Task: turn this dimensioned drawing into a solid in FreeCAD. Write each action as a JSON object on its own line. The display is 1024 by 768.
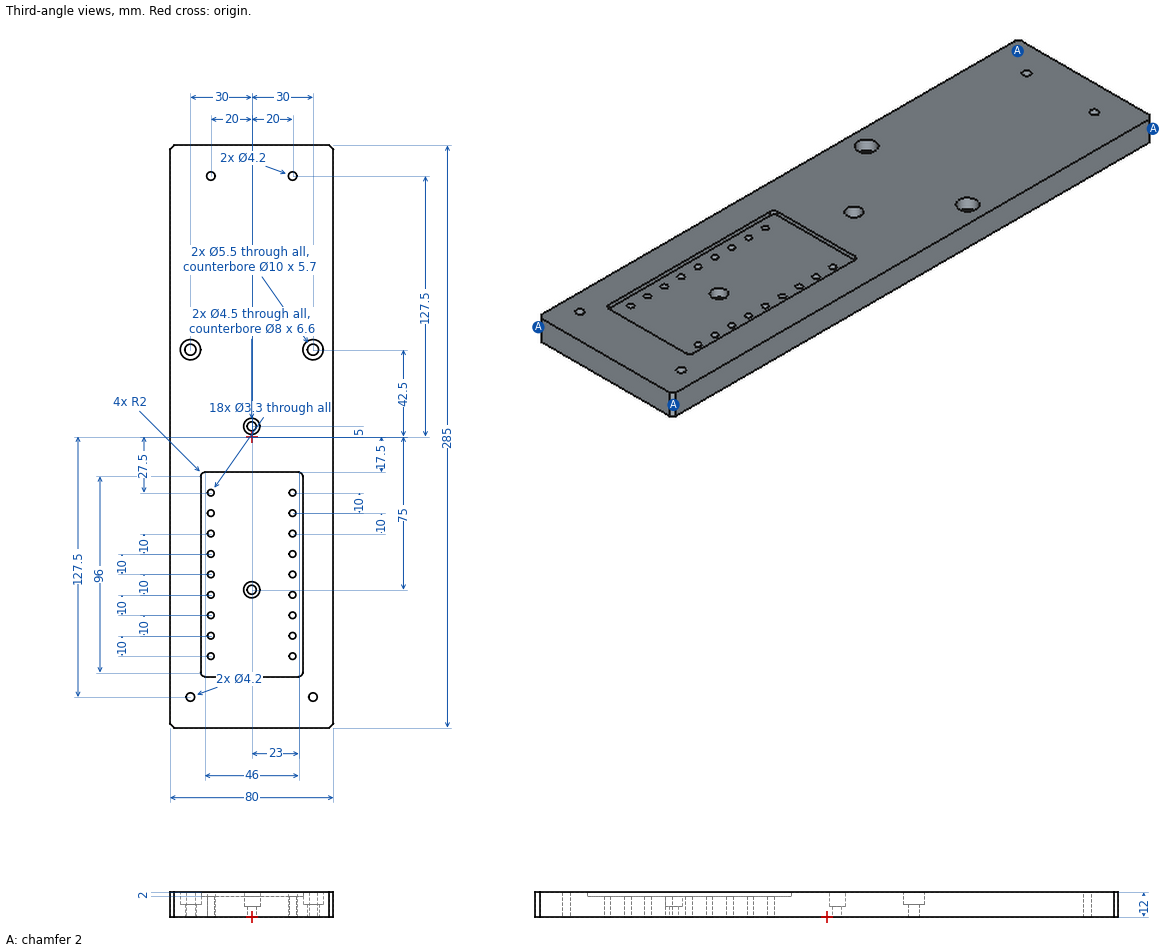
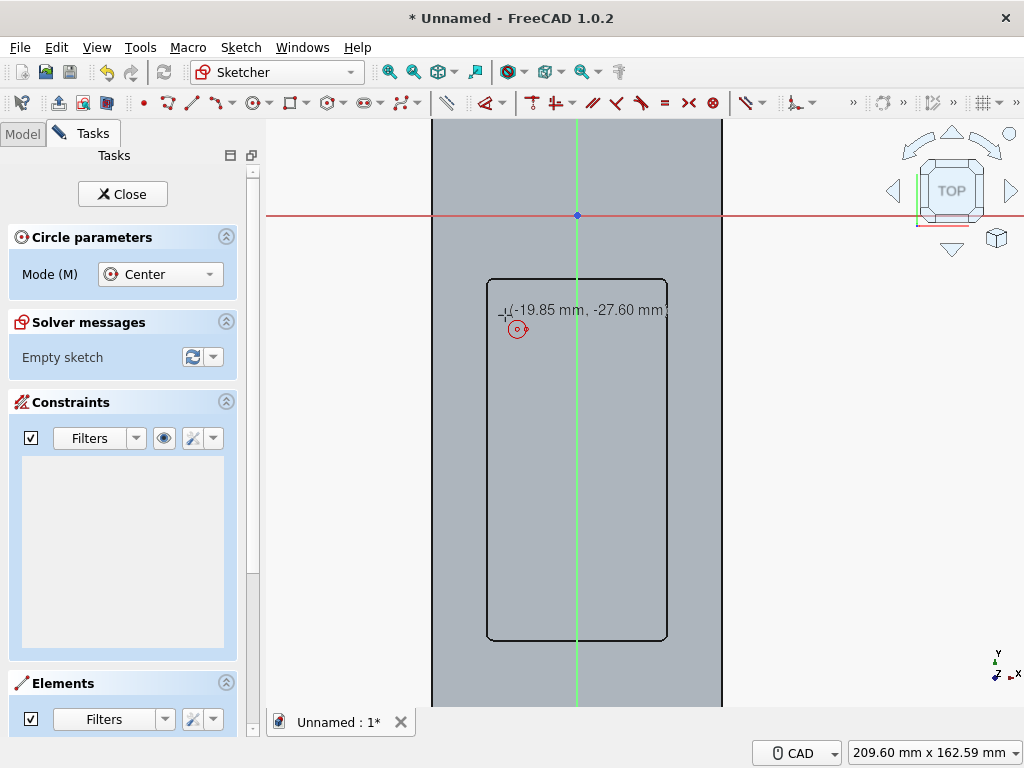
{"action": "left_click", "coordinate": [505, 315]}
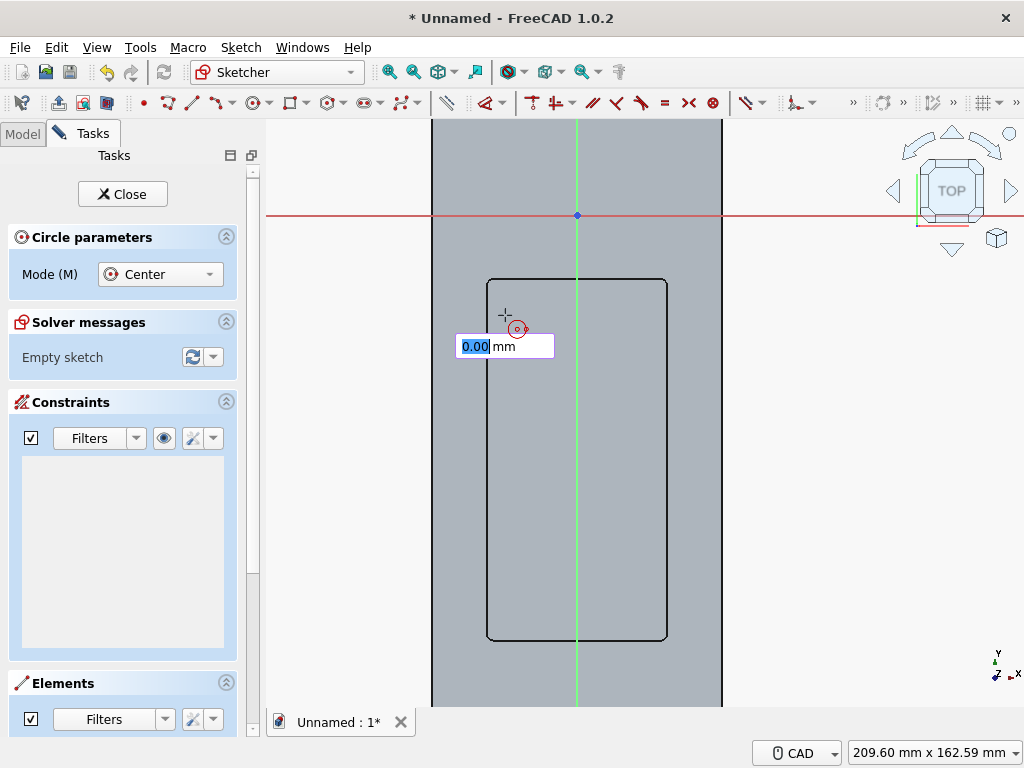
{"action": "scroll", "coordinate": [509, 311], "scroll_direction": "up", "scroll_amount": 5}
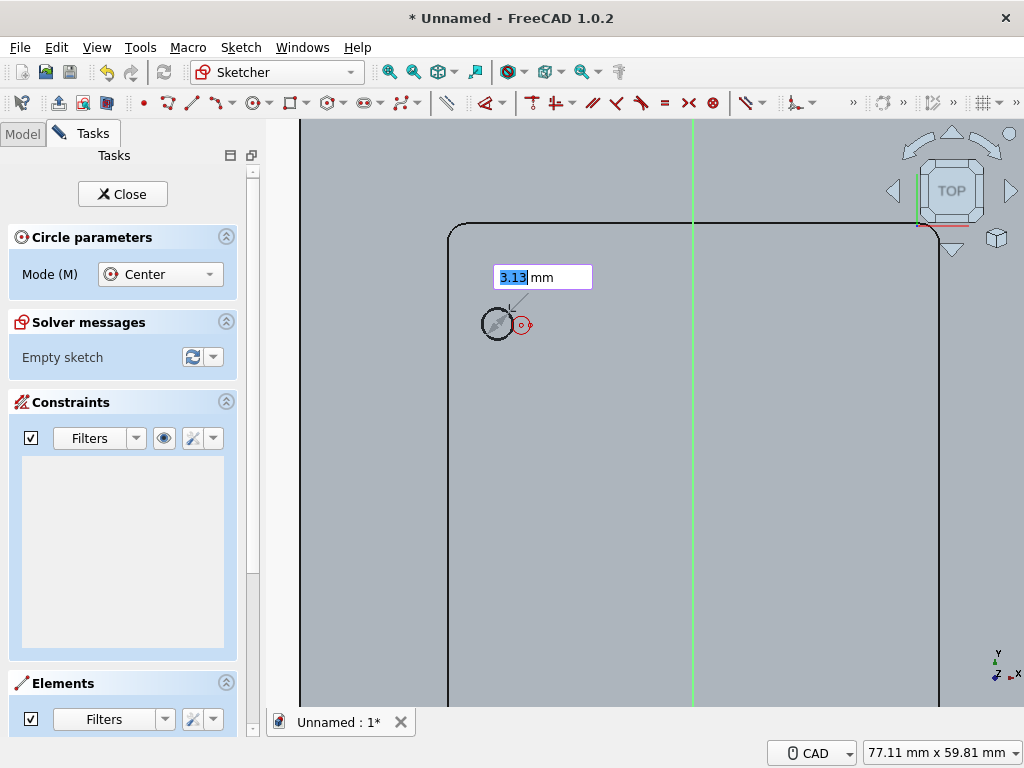
{"action": "left_click", "coordinate": [508, 310]}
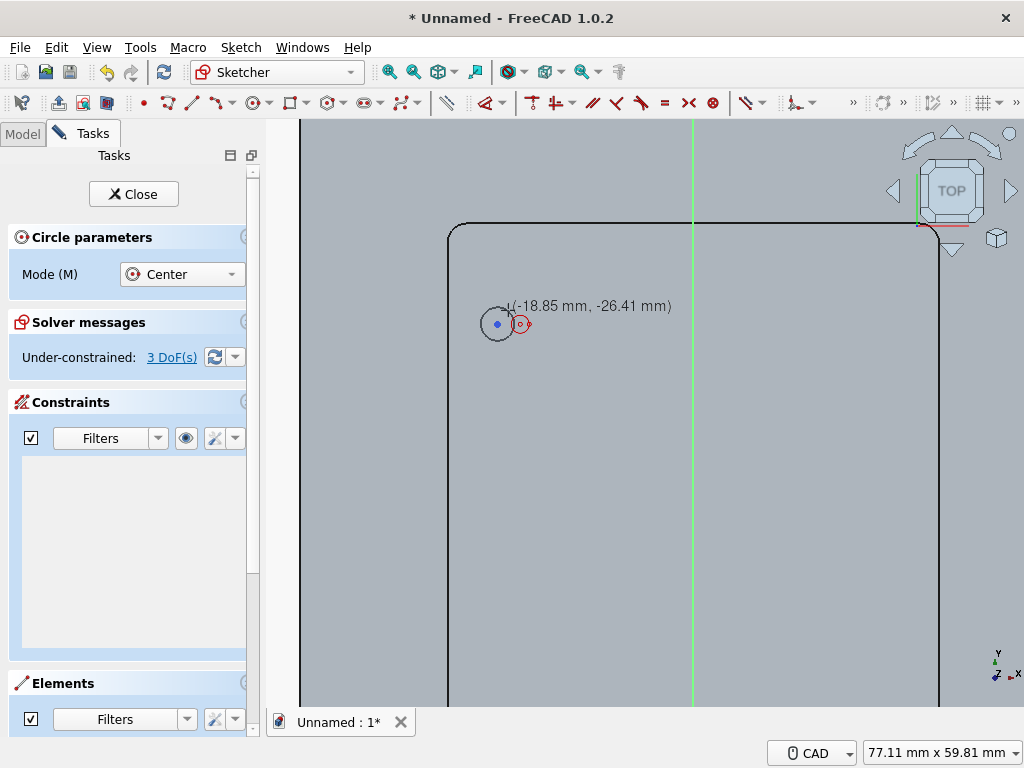
{"action": "scroll", "coordinate": [509, 311], "scroll_direction": "down", "scroll_amount": 5}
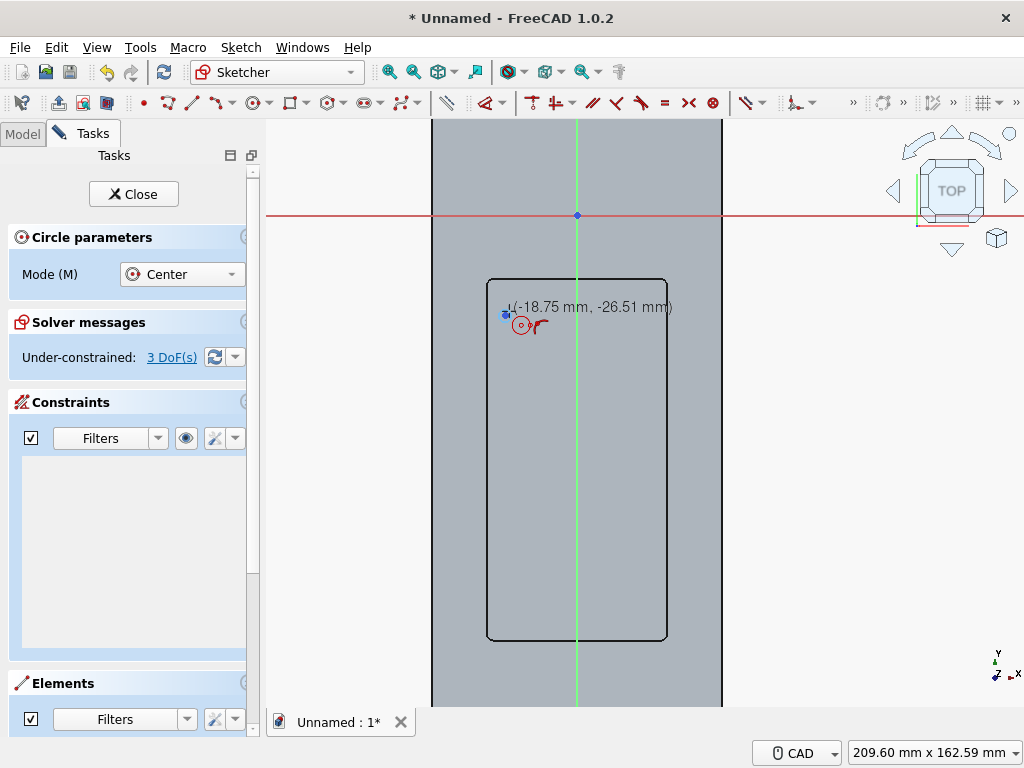
{"action": "scroll", "coordinate": [649, 315], "scroll_direction": "up", "scroll_amount": 7}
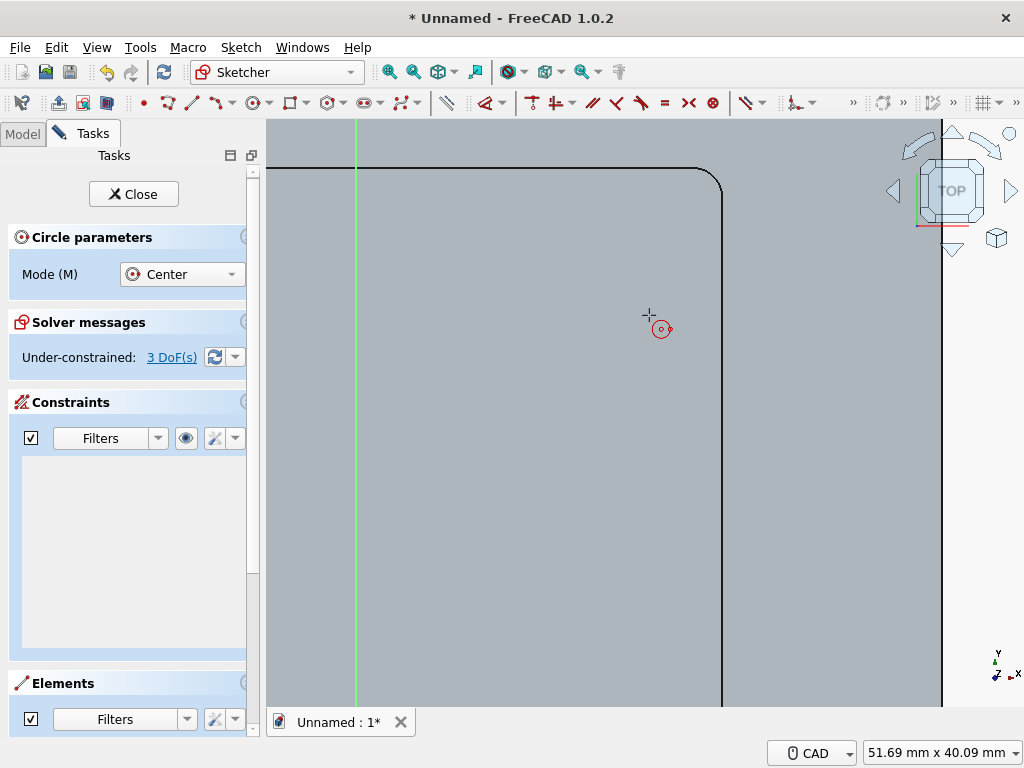
{"action": "scroll", "coordinate": [649, 315], "scroll_direction": "down", "scroll_amount": 7}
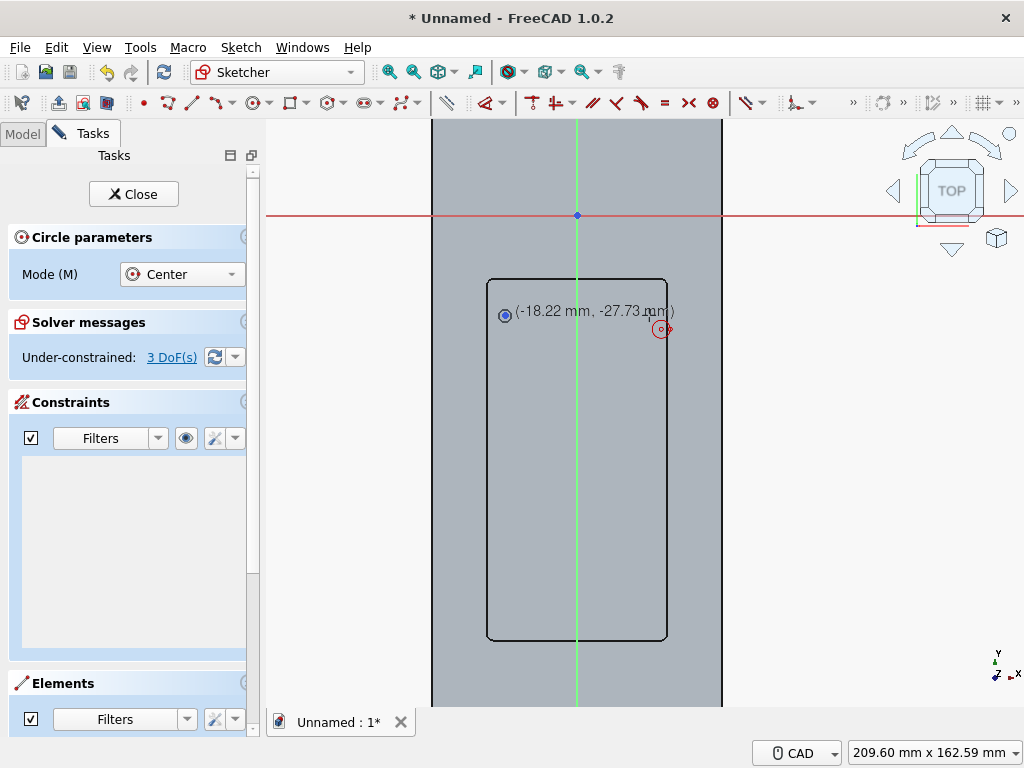
{"action": "left_click", "coordinate": [649, 315]}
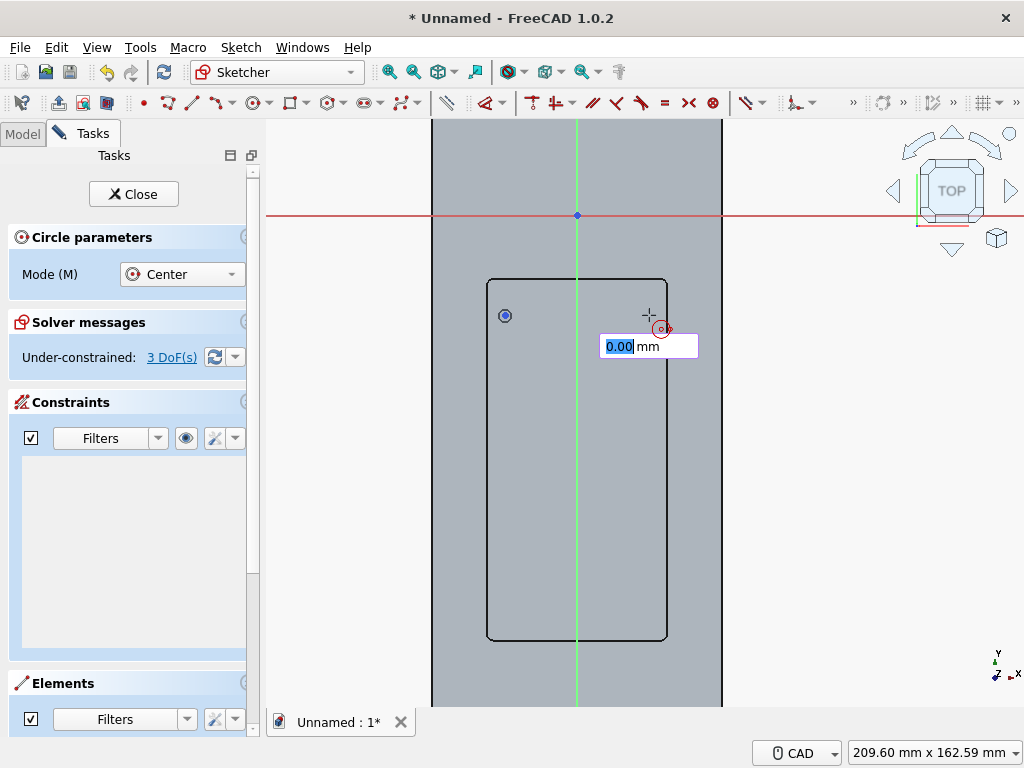
{"action": "scroll", "coordinate": [654, 311], "scroll_direction": "up", "scroll_amount": 5}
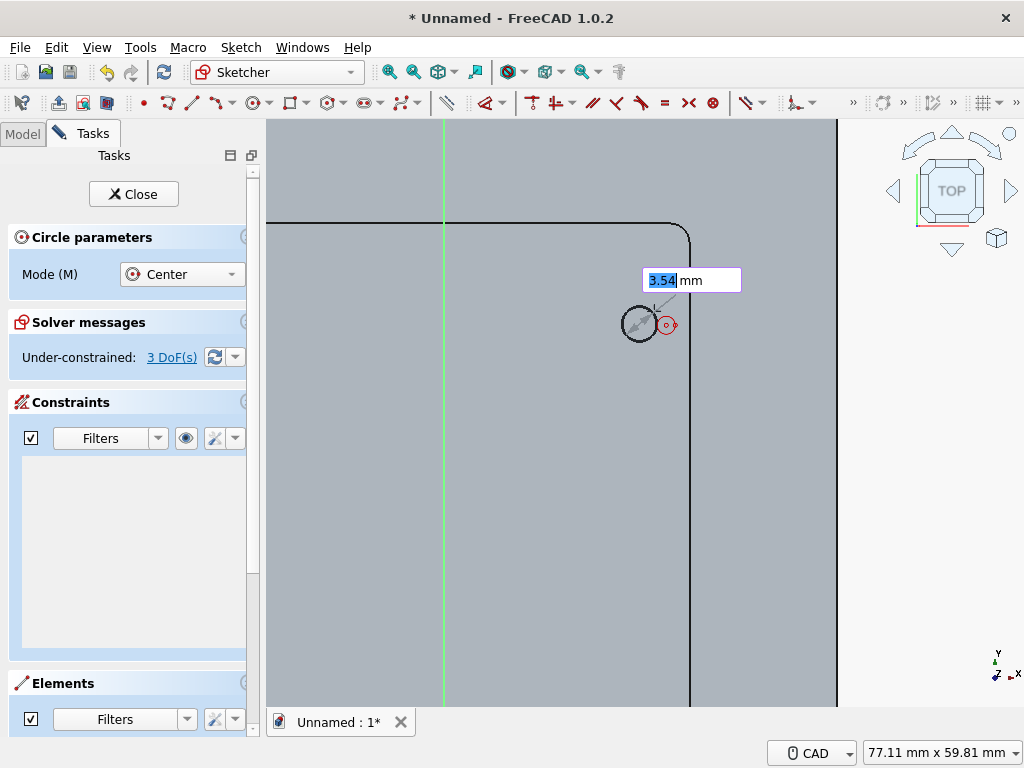
{"action": "left_click", "coordinate": [652, 310]}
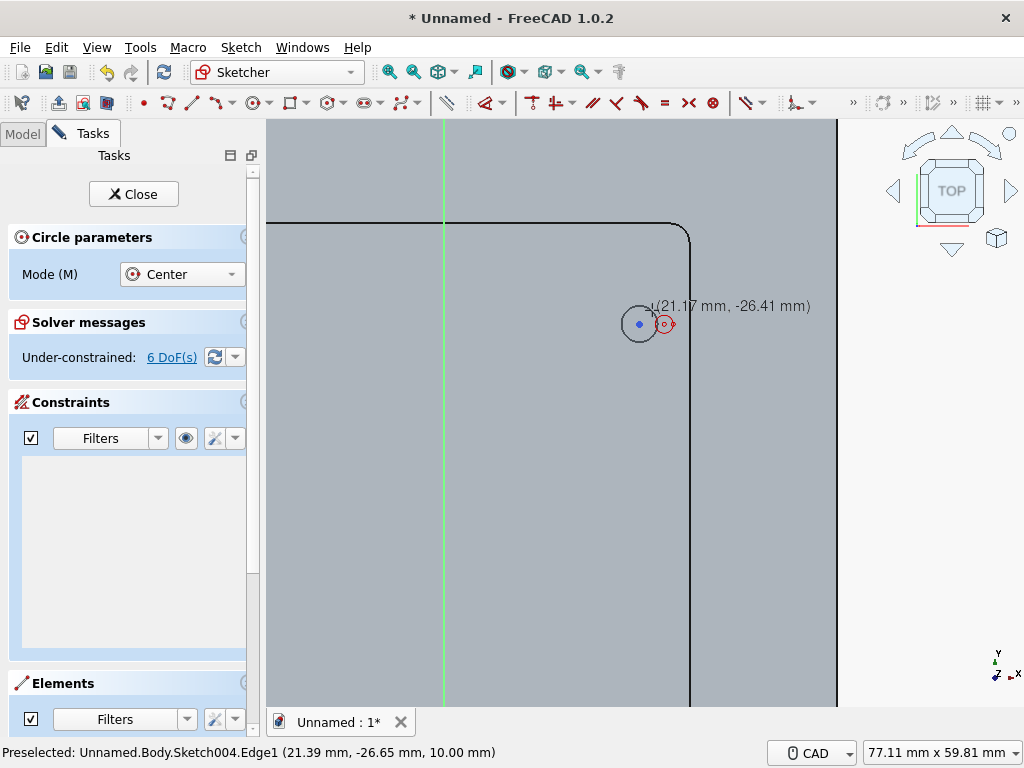
{"action": "scroll", "coordinate": [640, 420], "scroll_direction": "up", "scroll_amount": 2}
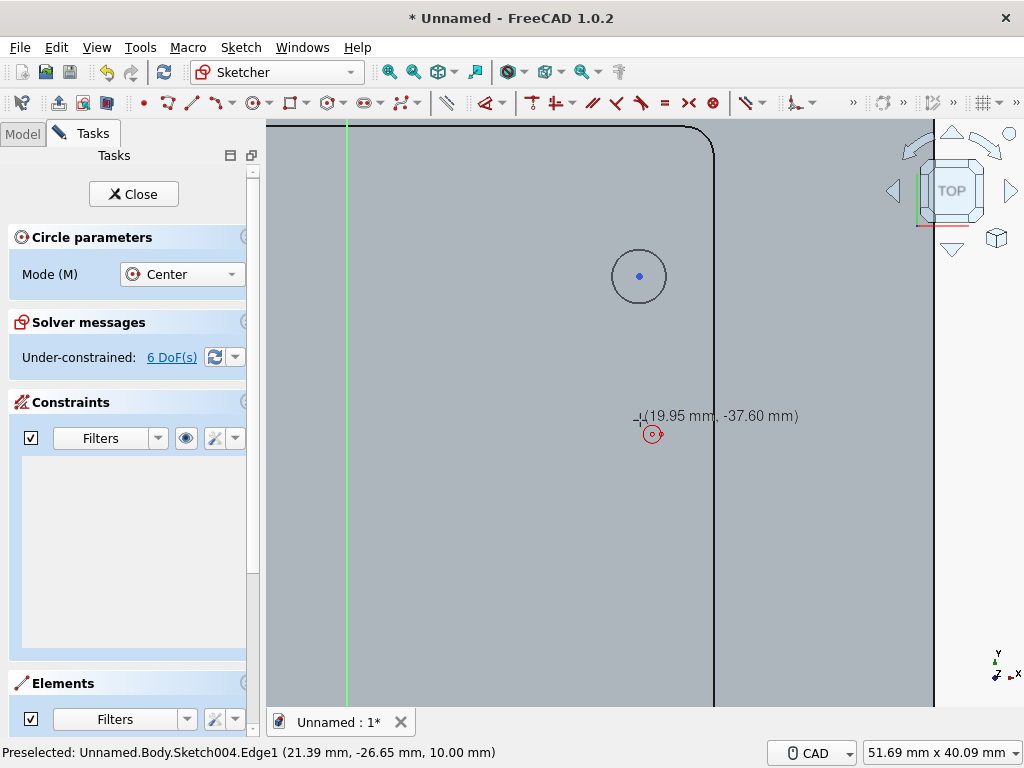
{"action": "scroll", "coordinate": [652, 329], "scroll_direction": "down", "scroll_amount": 7}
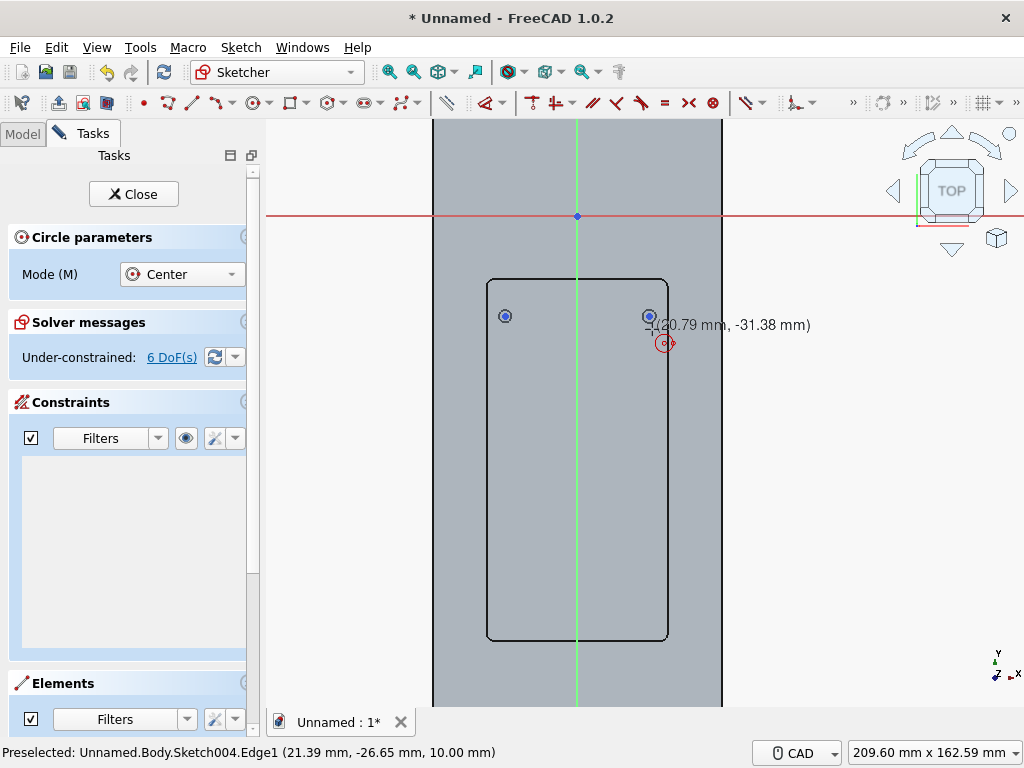
{"action": "left_click", "coordinate": [650, 352]}